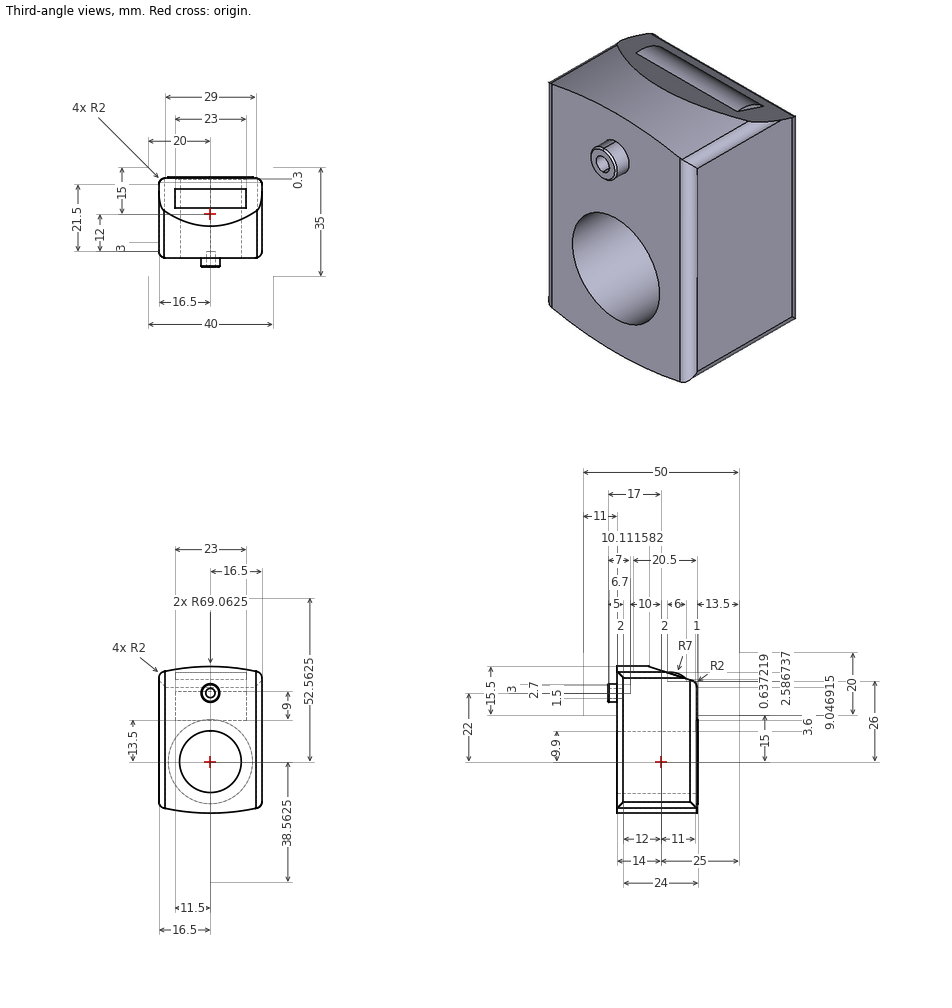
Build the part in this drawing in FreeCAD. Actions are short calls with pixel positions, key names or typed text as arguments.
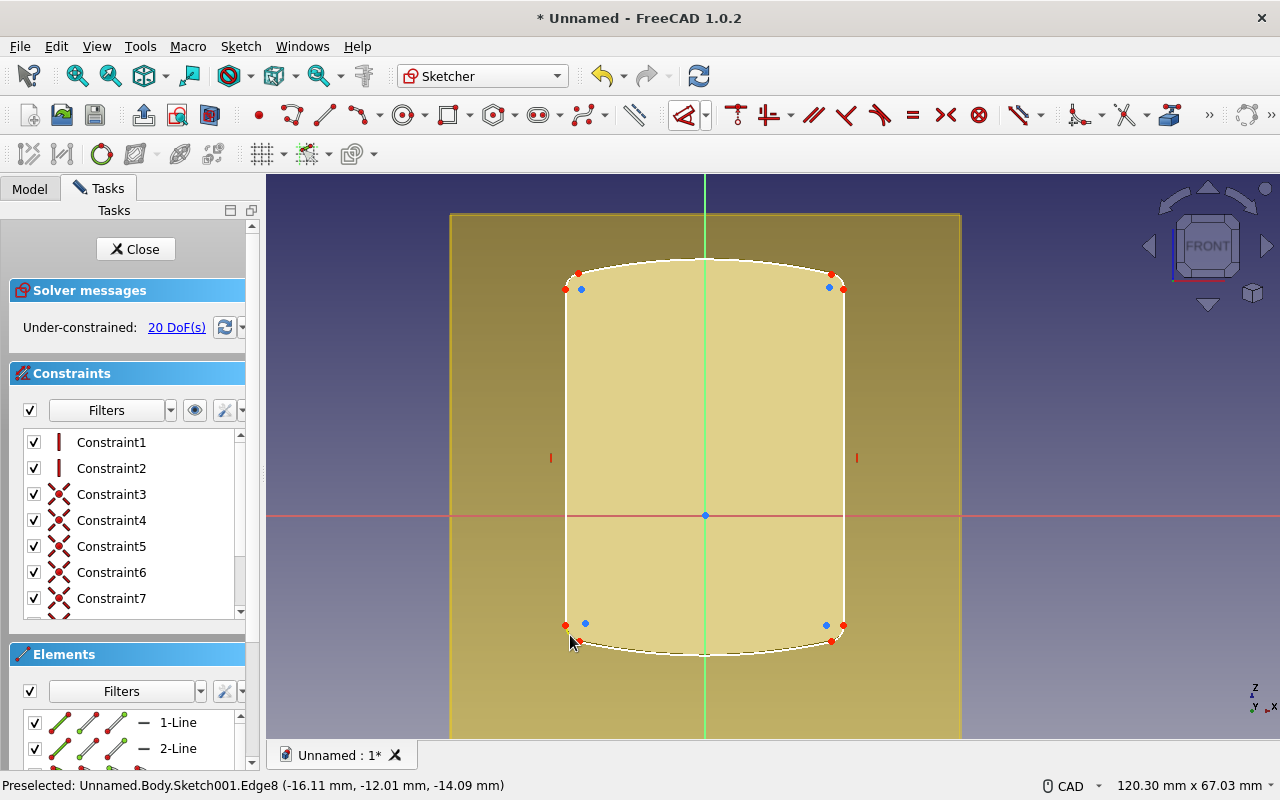
click(566, 559)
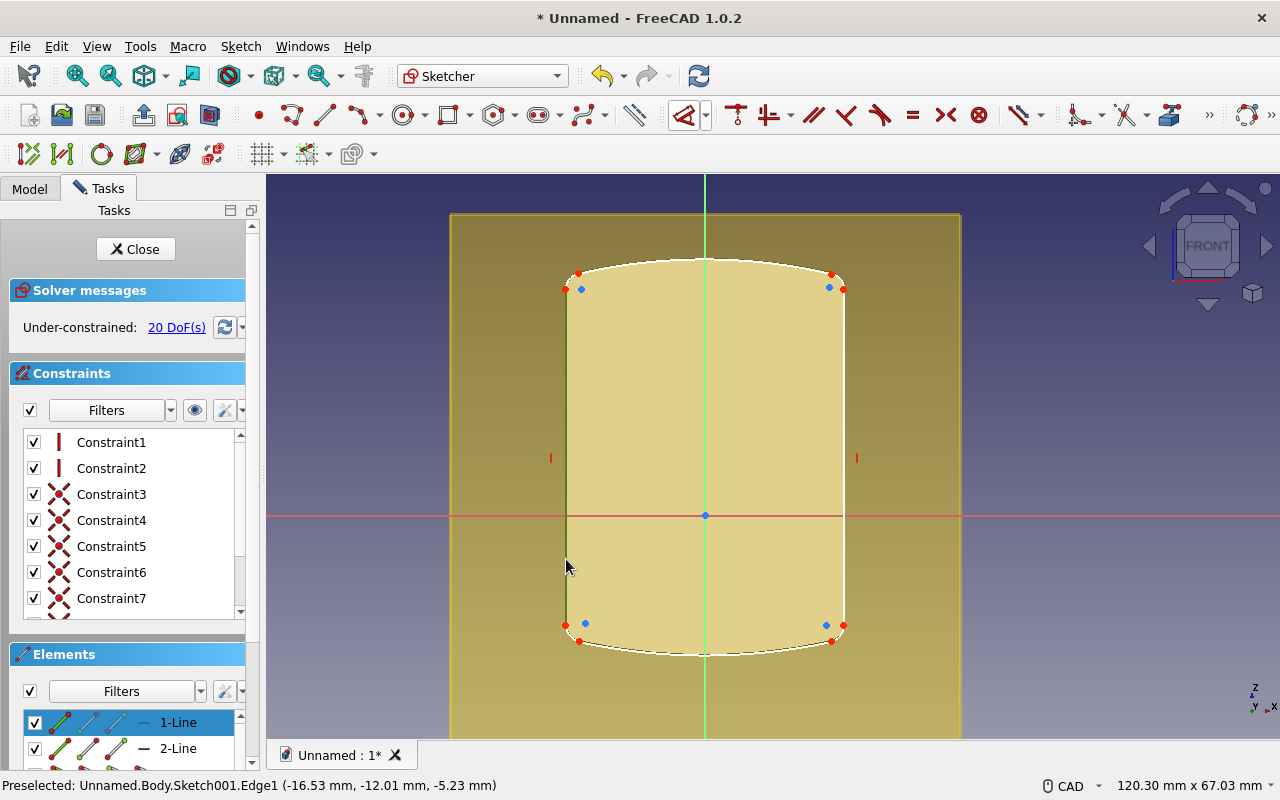
scroll(569, 279, up, 2)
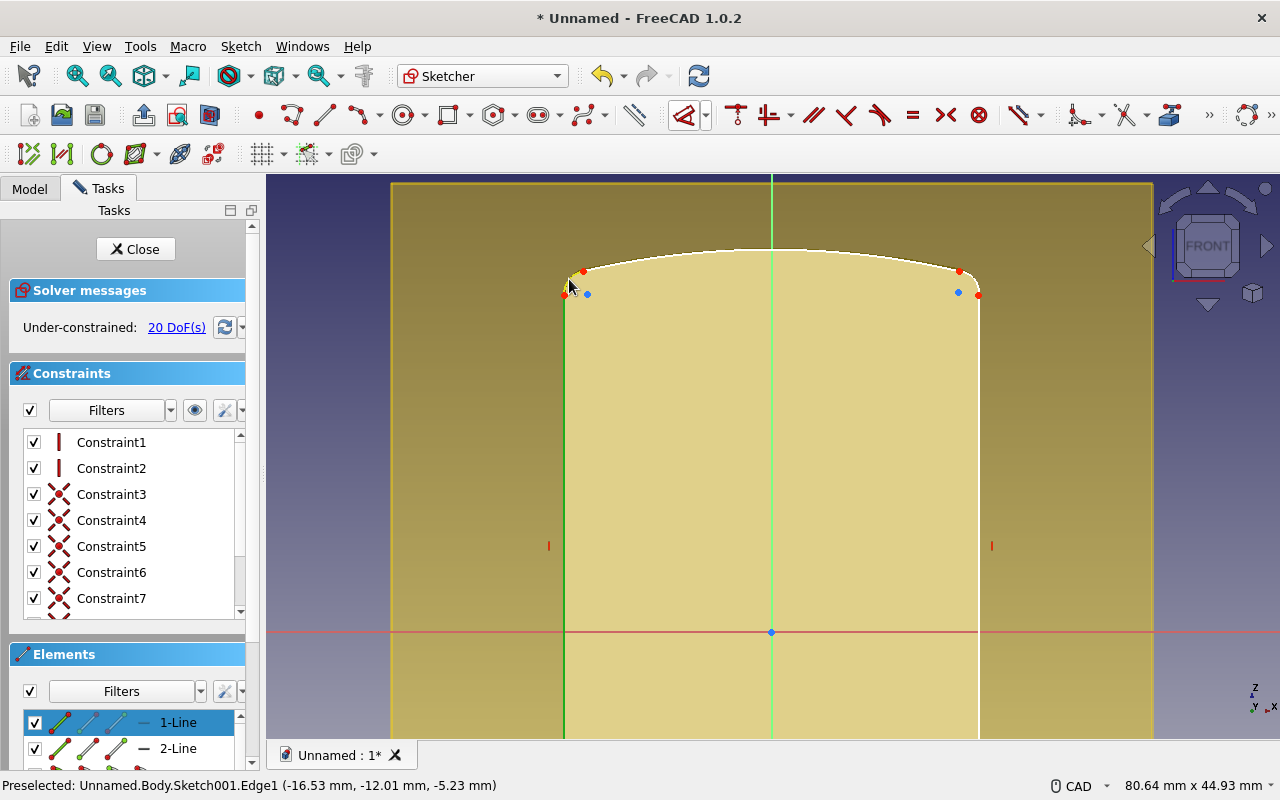
click(569, 279)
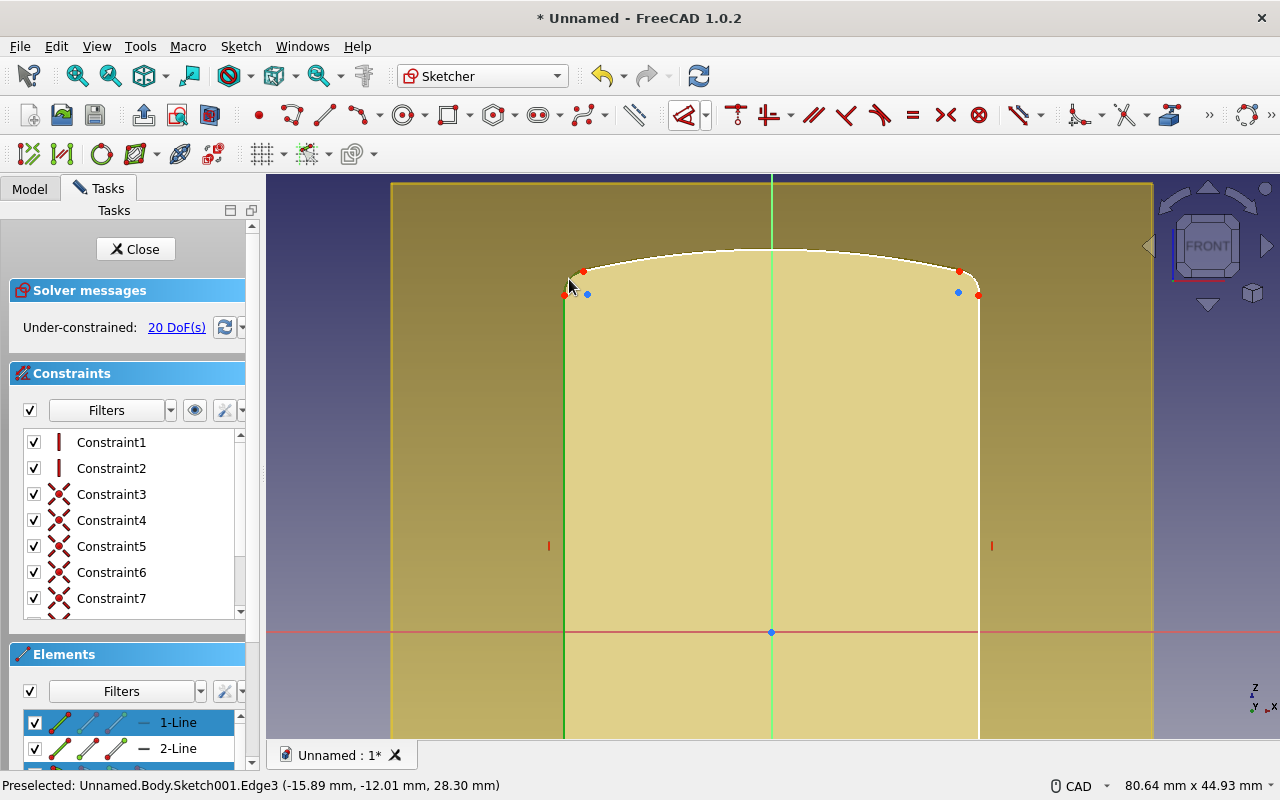
click(880, 116)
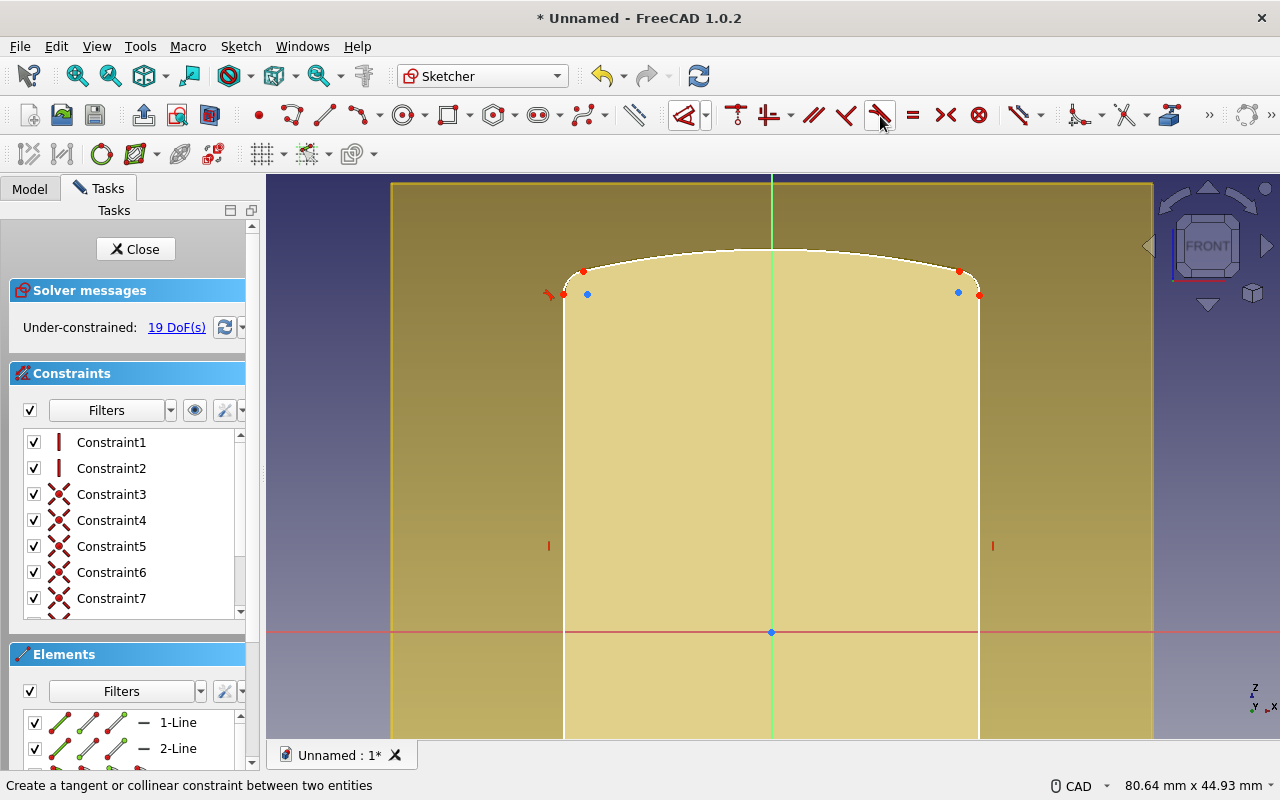
click(564, 646)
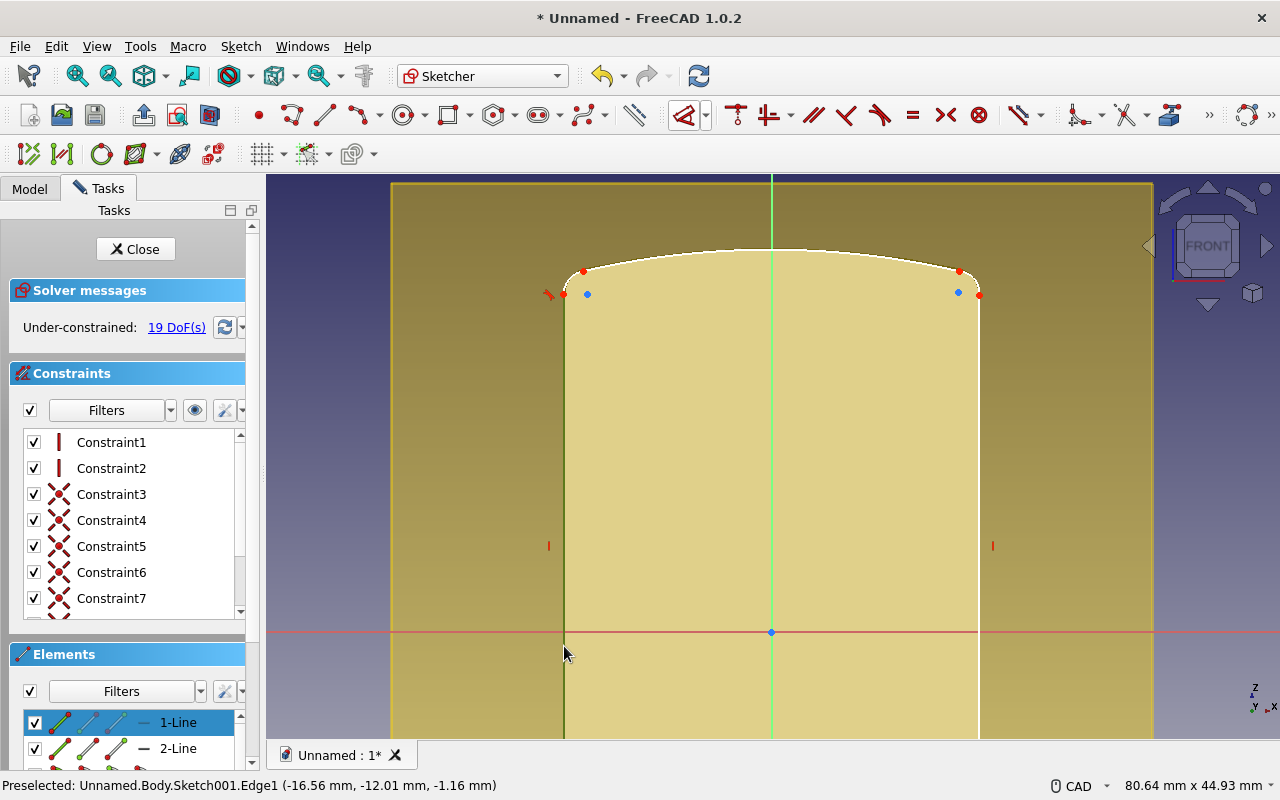
scroll(567, 278, down, 2)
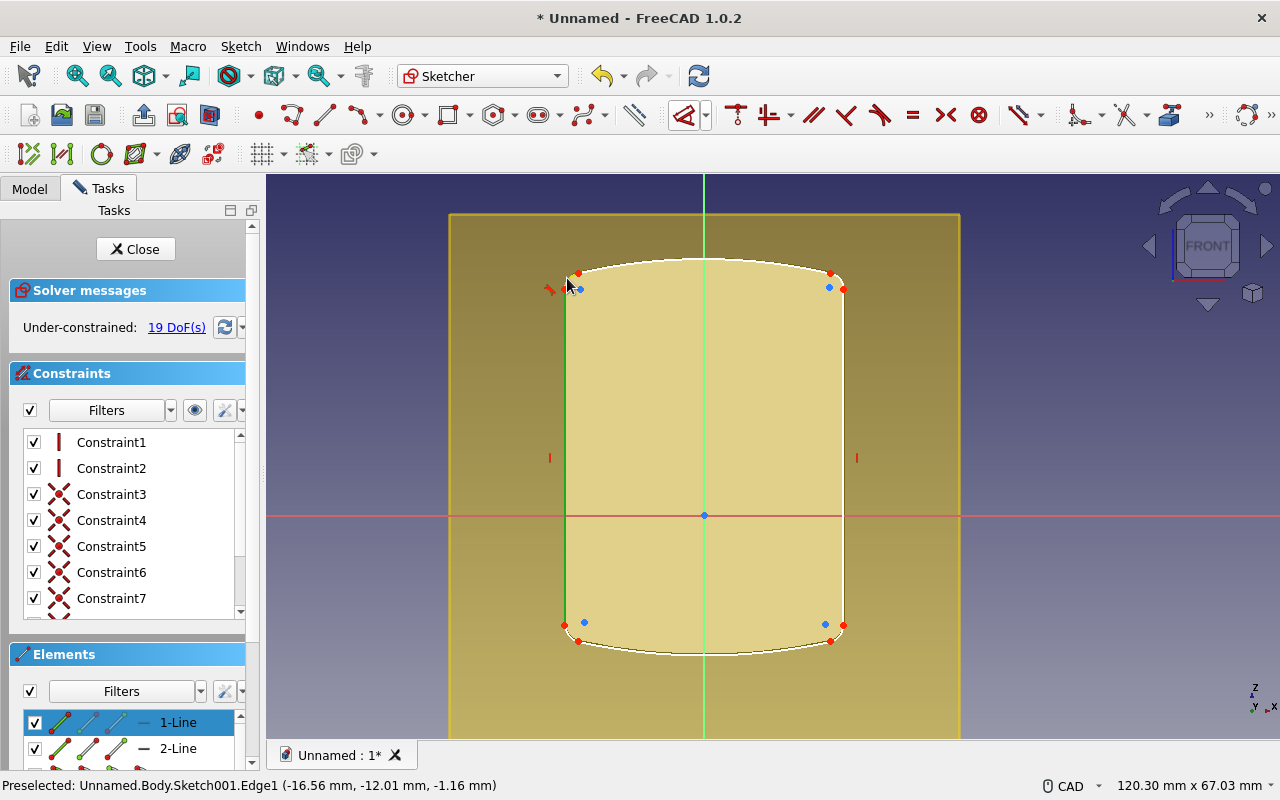
scroll(567, 632, up, 4)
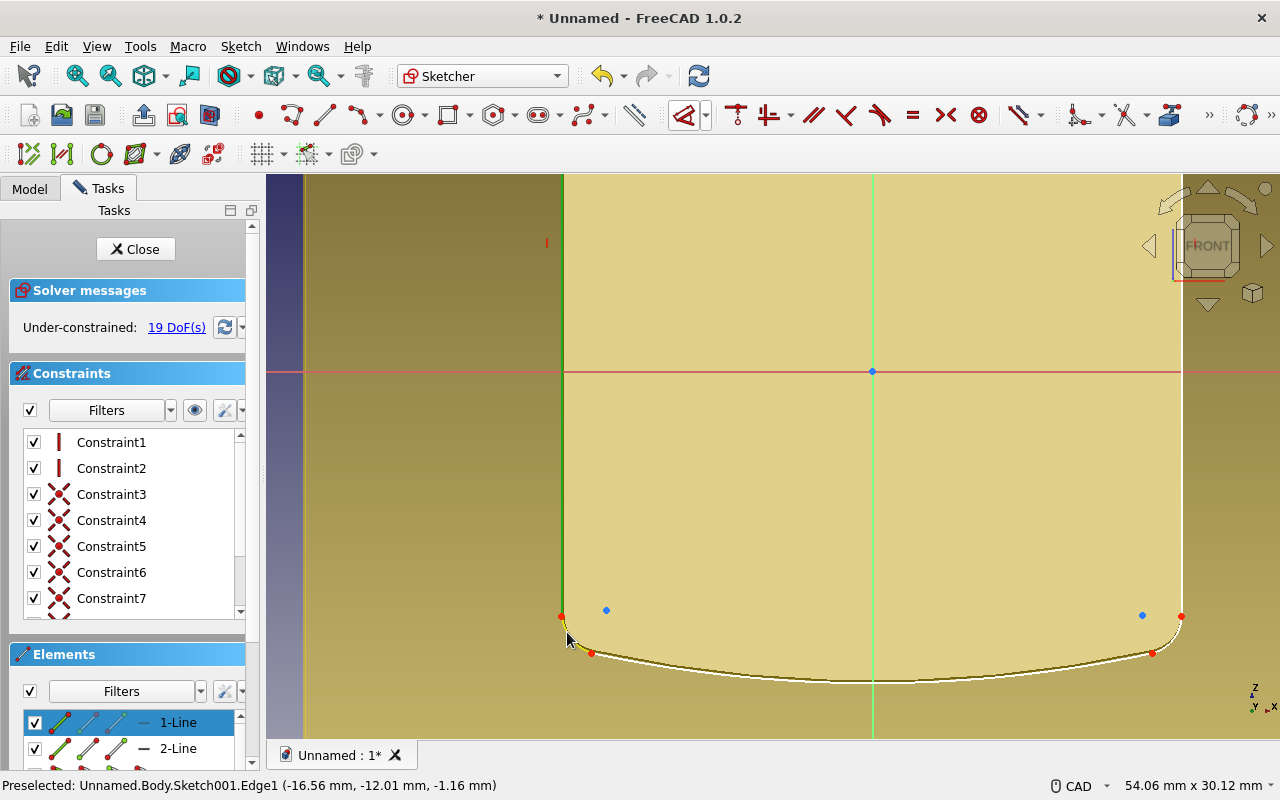
click(566, 631)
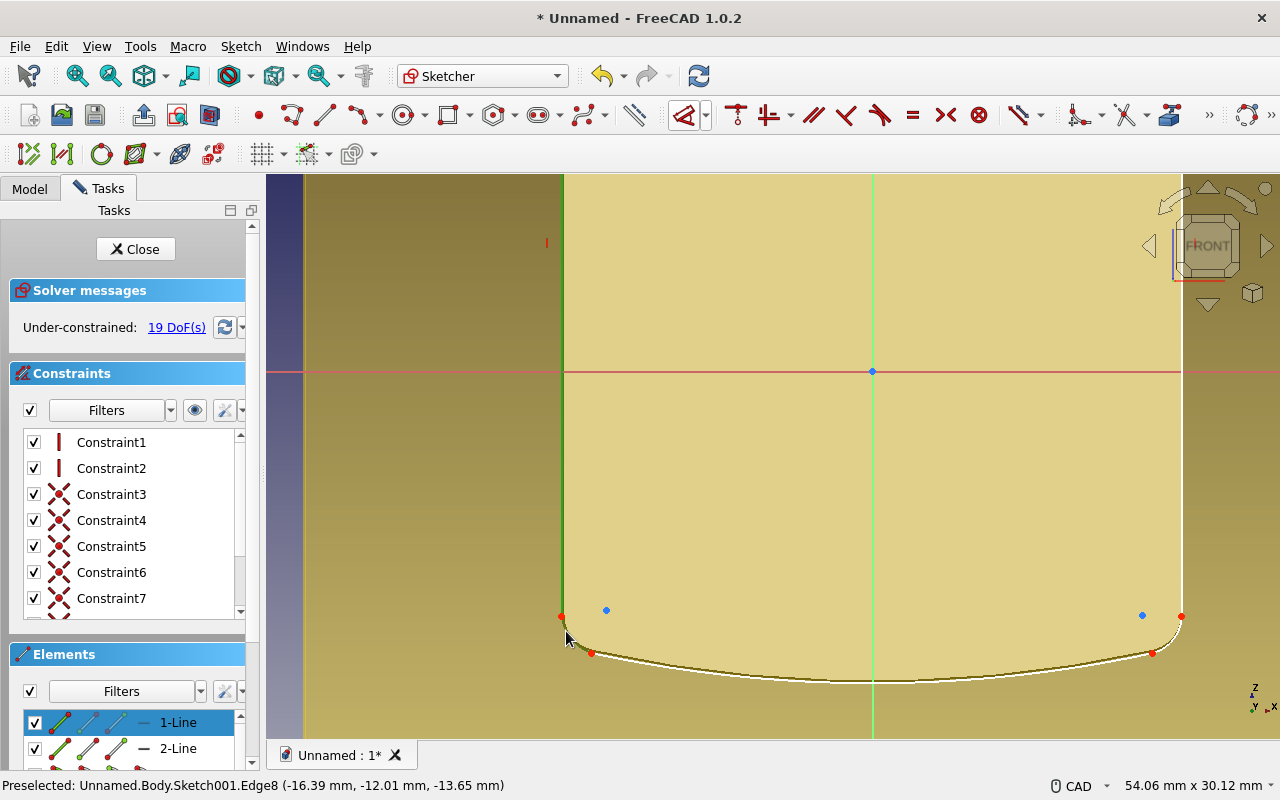
click(880, 116)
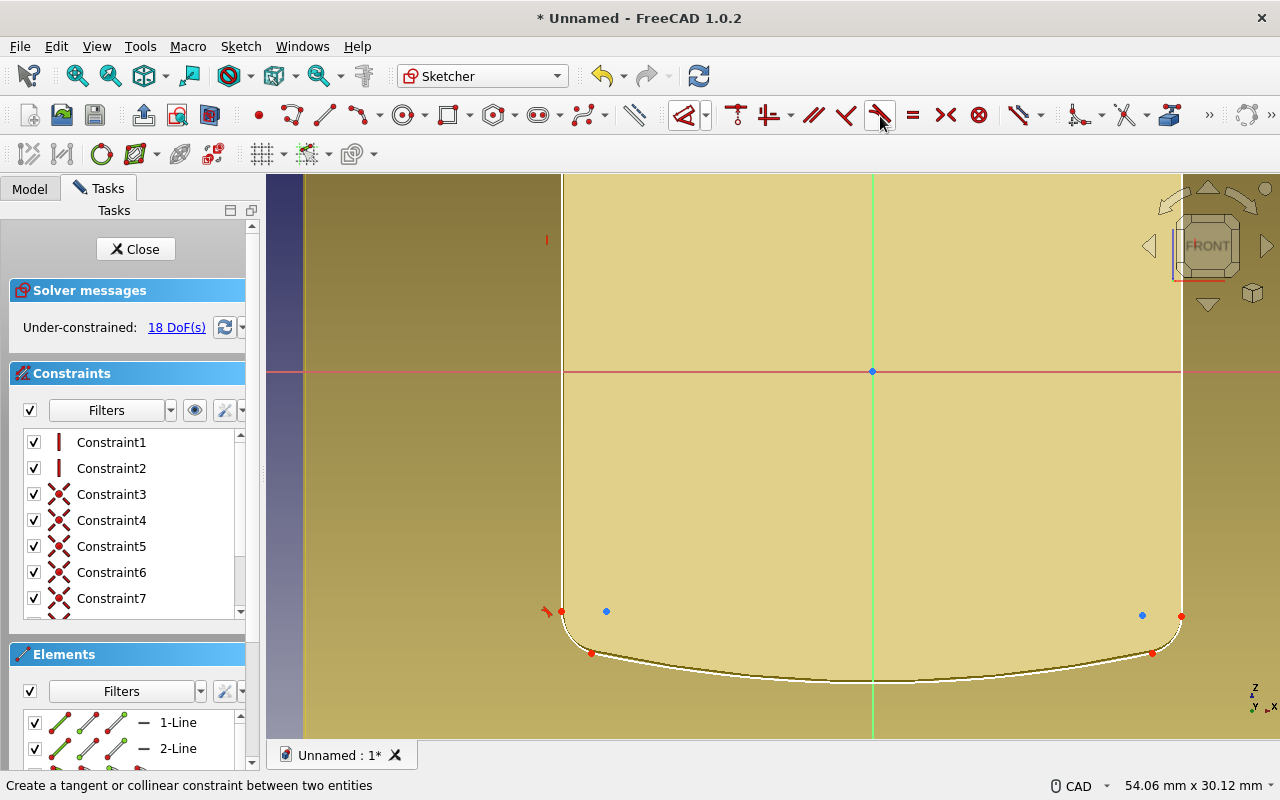
scroll(567, 633, down, 4)